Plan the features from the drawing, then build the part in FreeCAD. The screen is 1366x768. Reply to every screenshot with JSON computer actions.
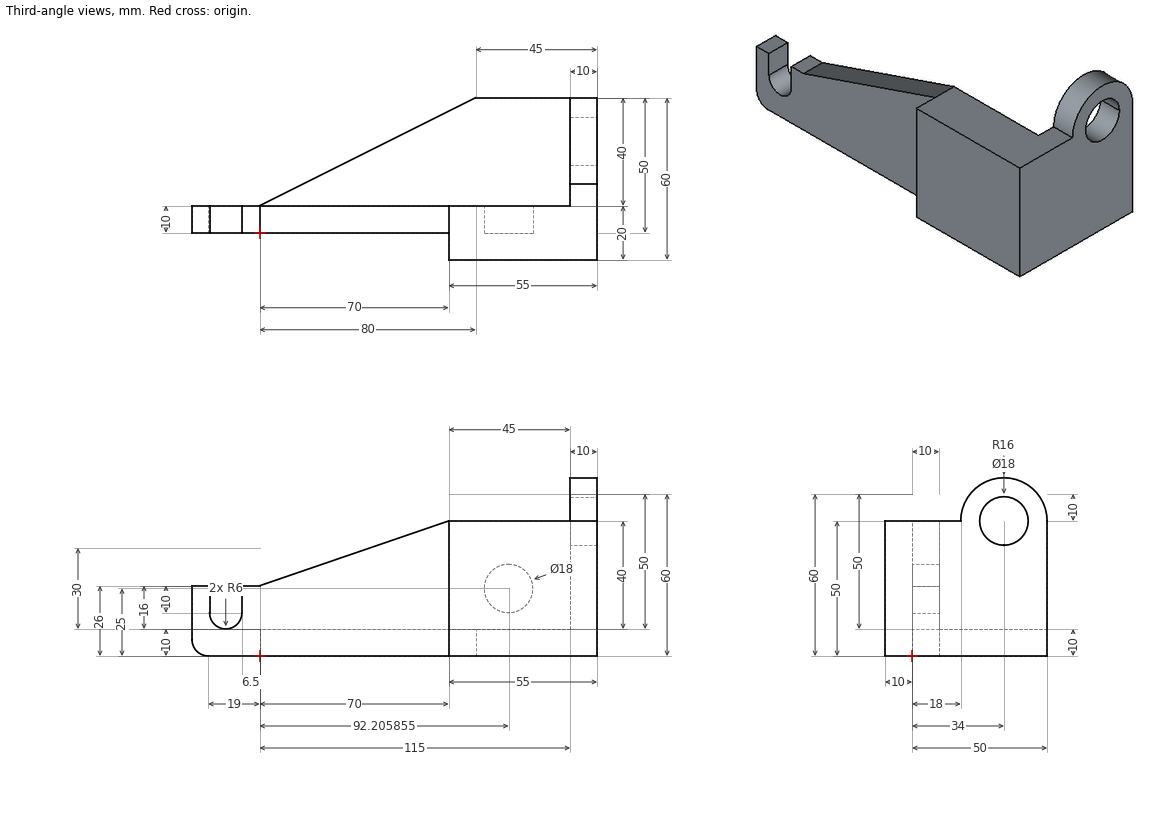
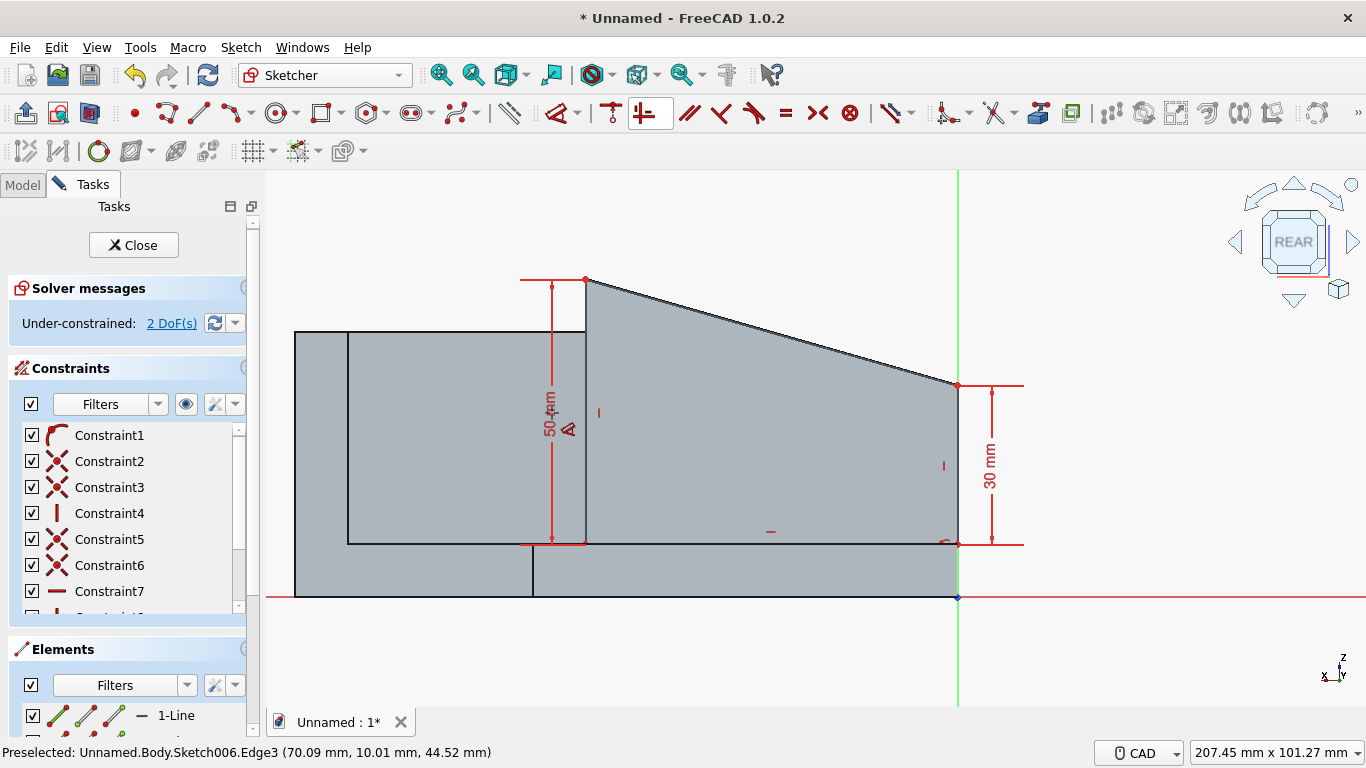
{"action": "left_click", "coordinate": [697, 545]}
{"action": "left_click", "coordinate": [772, 579]}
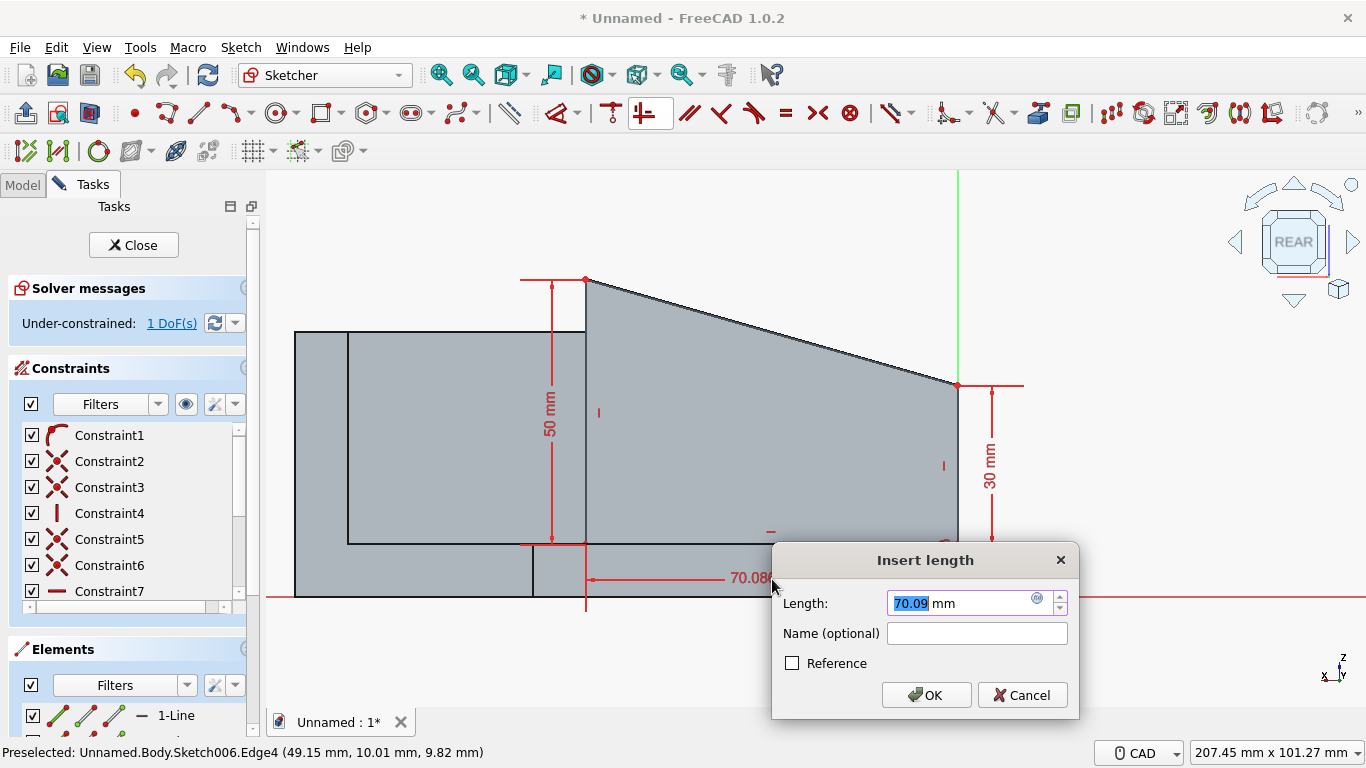
{"action": "type", "text": "70"}
{"action": "key", "text": "Return"}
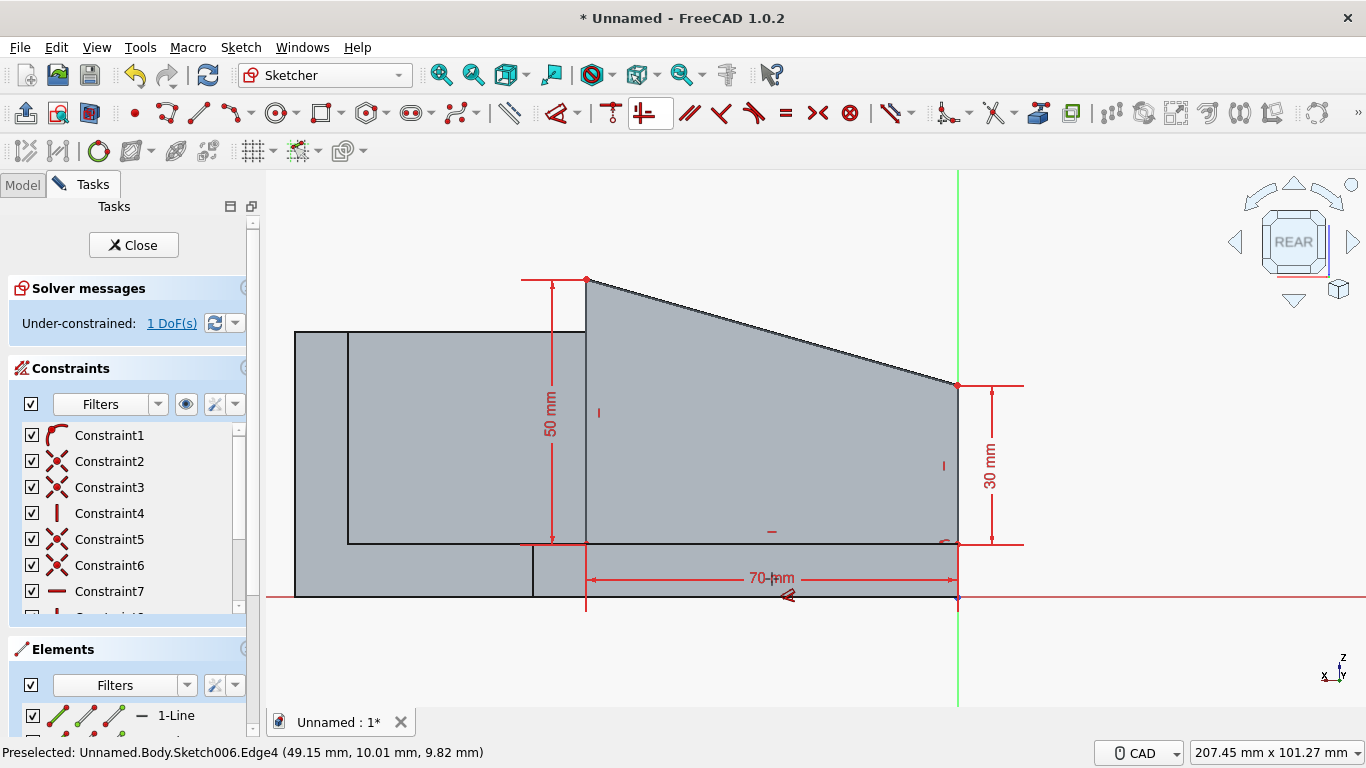
{"action": "left_click", "coordinate": [958, 545]}
{"action": "left_click", "coordinate": [992, 571]}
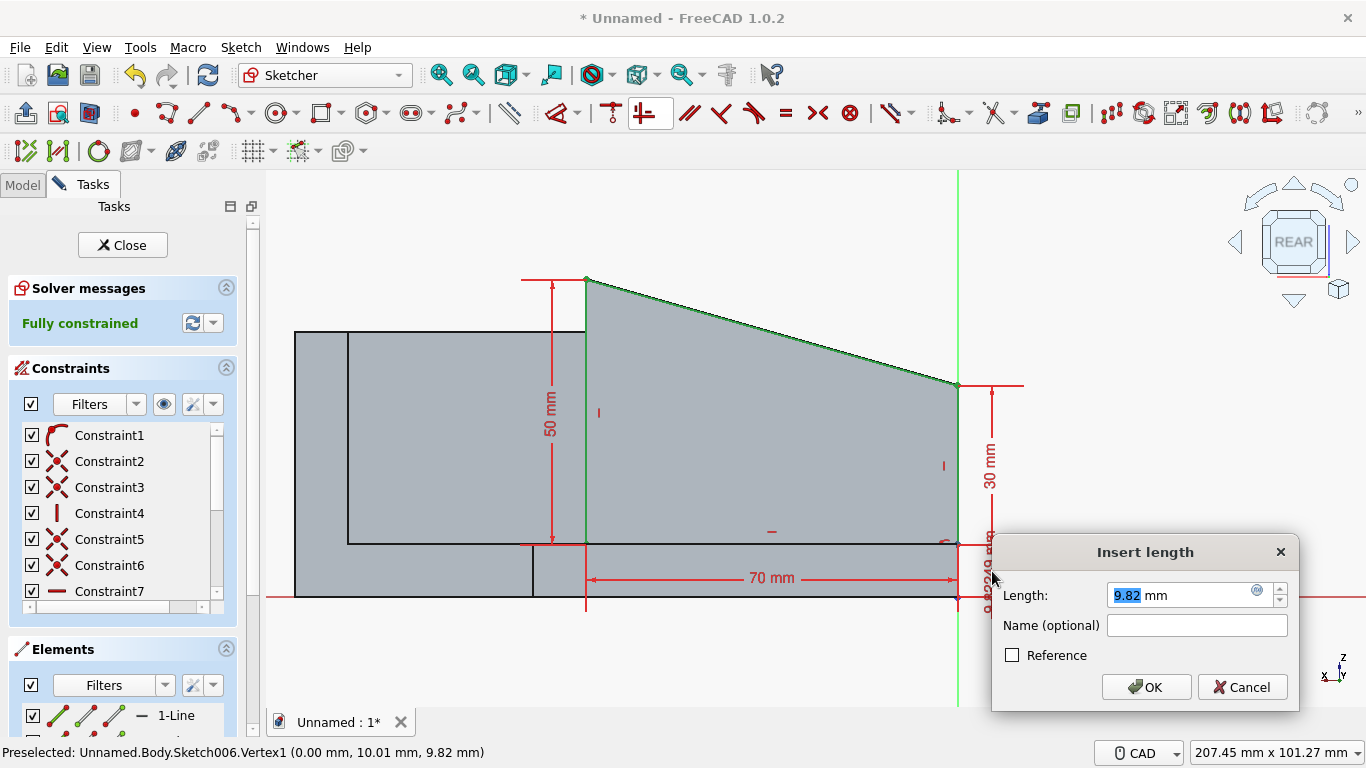
{"action": "type", "text": "10"}
{"action": "key", "text": "Return"}
{"action": "key", "text": "Escape"}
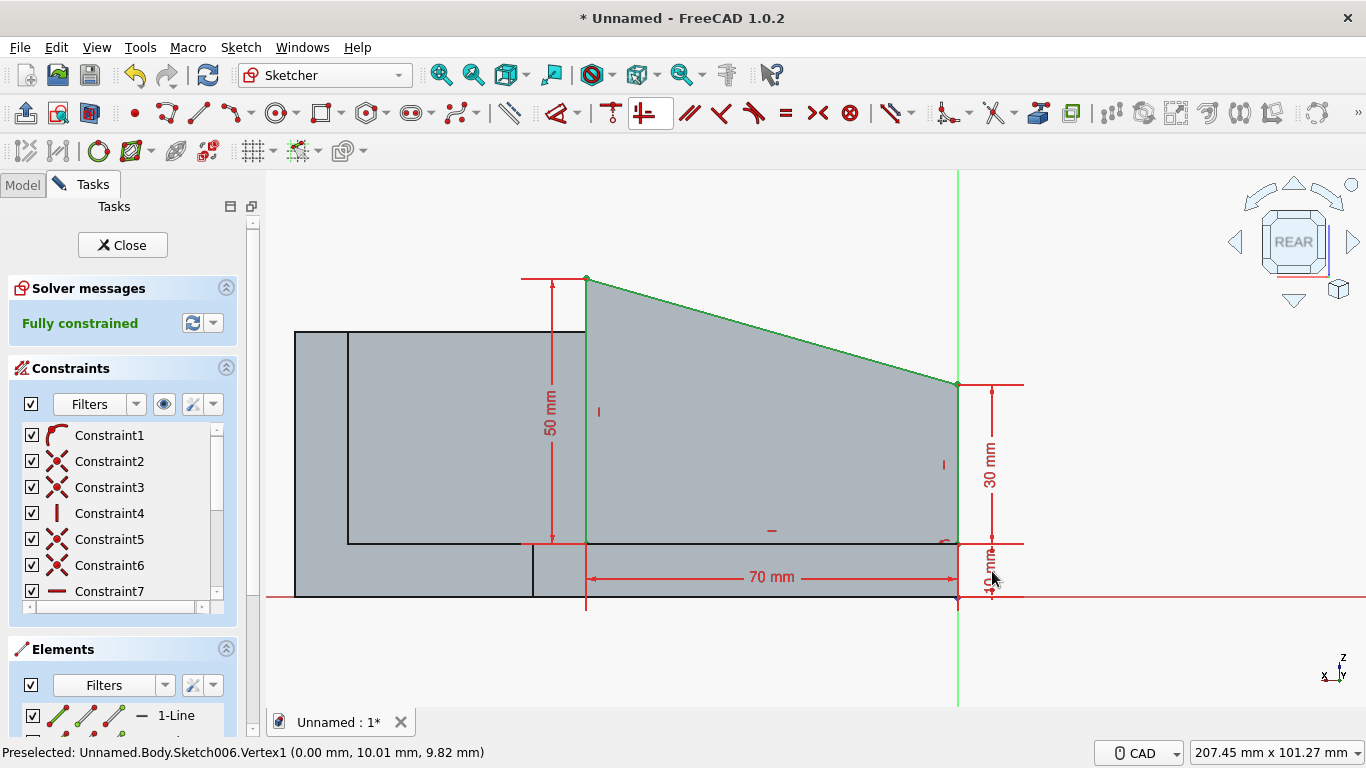
{"action": "left_click", "coordinate": [123, 245]}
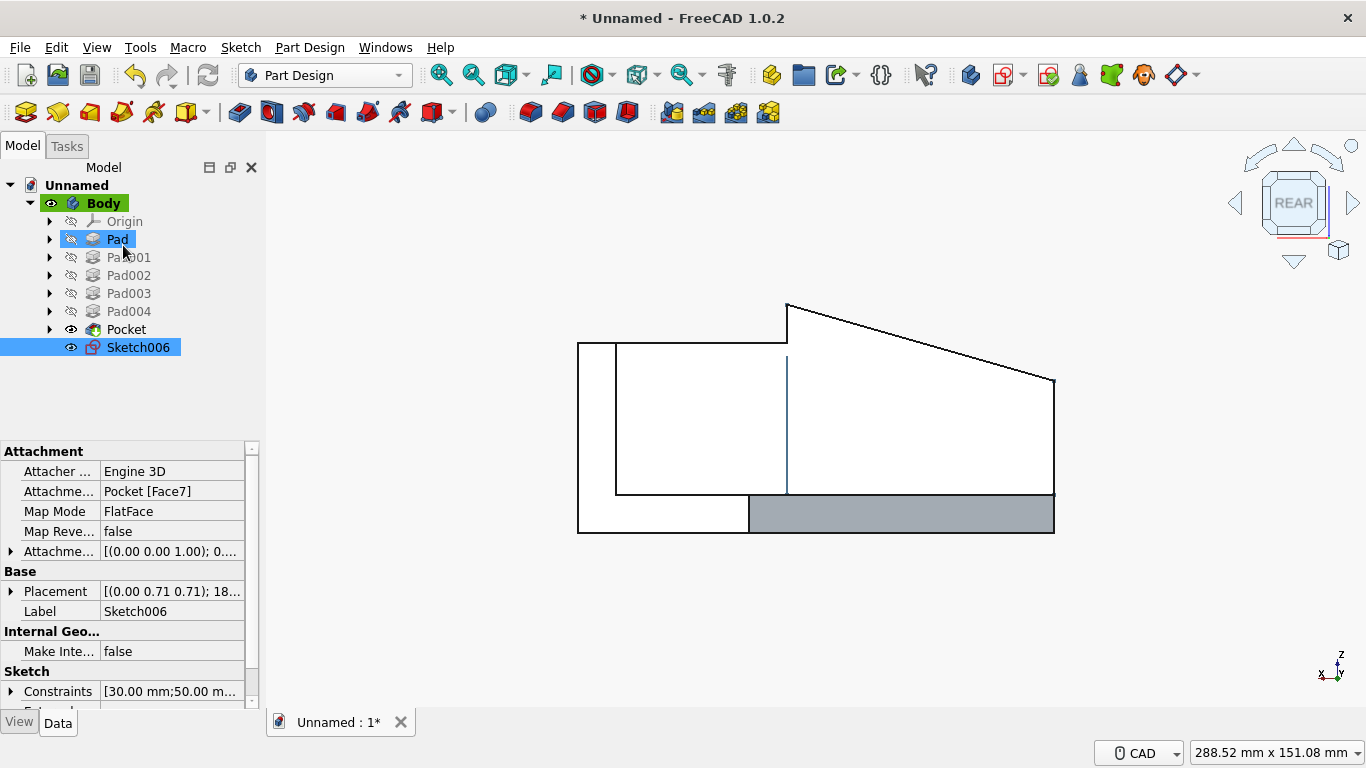
{"action": "left_click", "coordinate": [240, 112]}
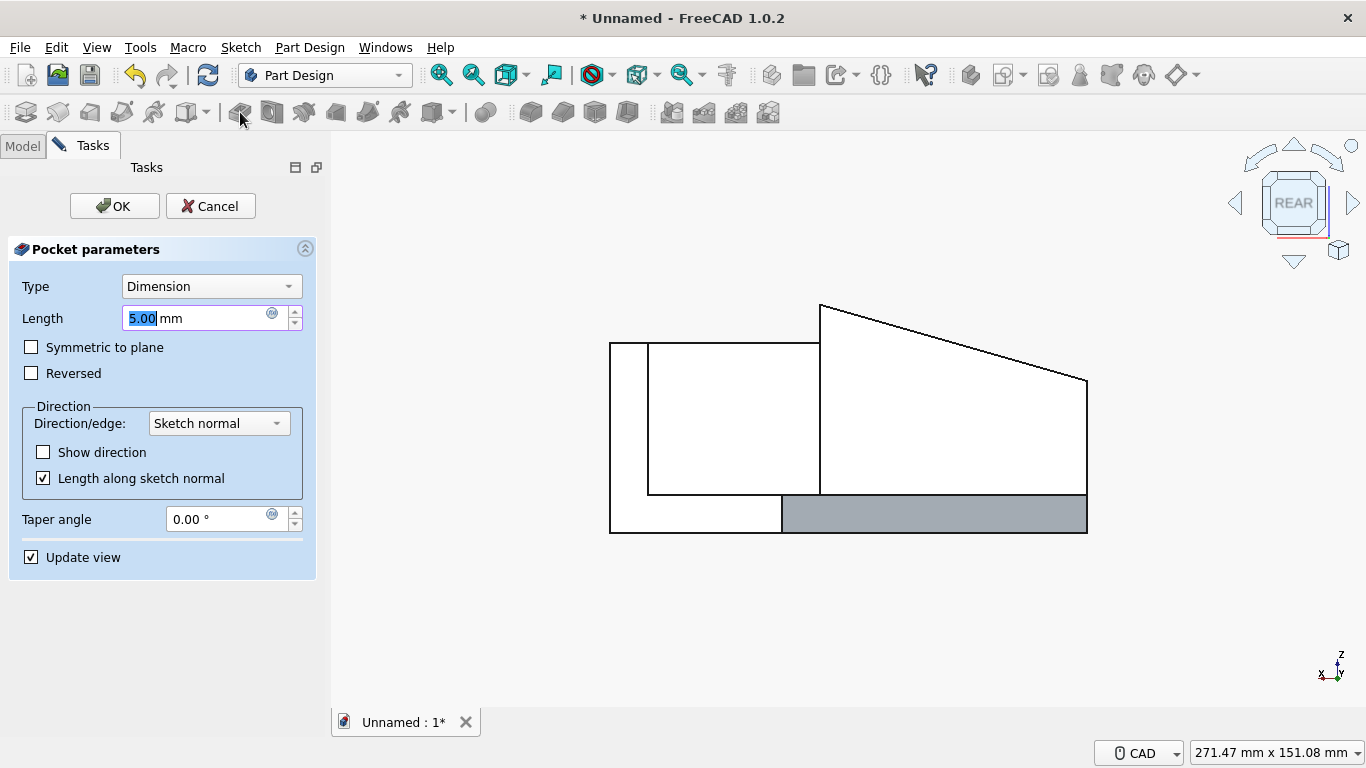
{"action": "type", "text": "10"}
{"action": "key", "text": "Tab"}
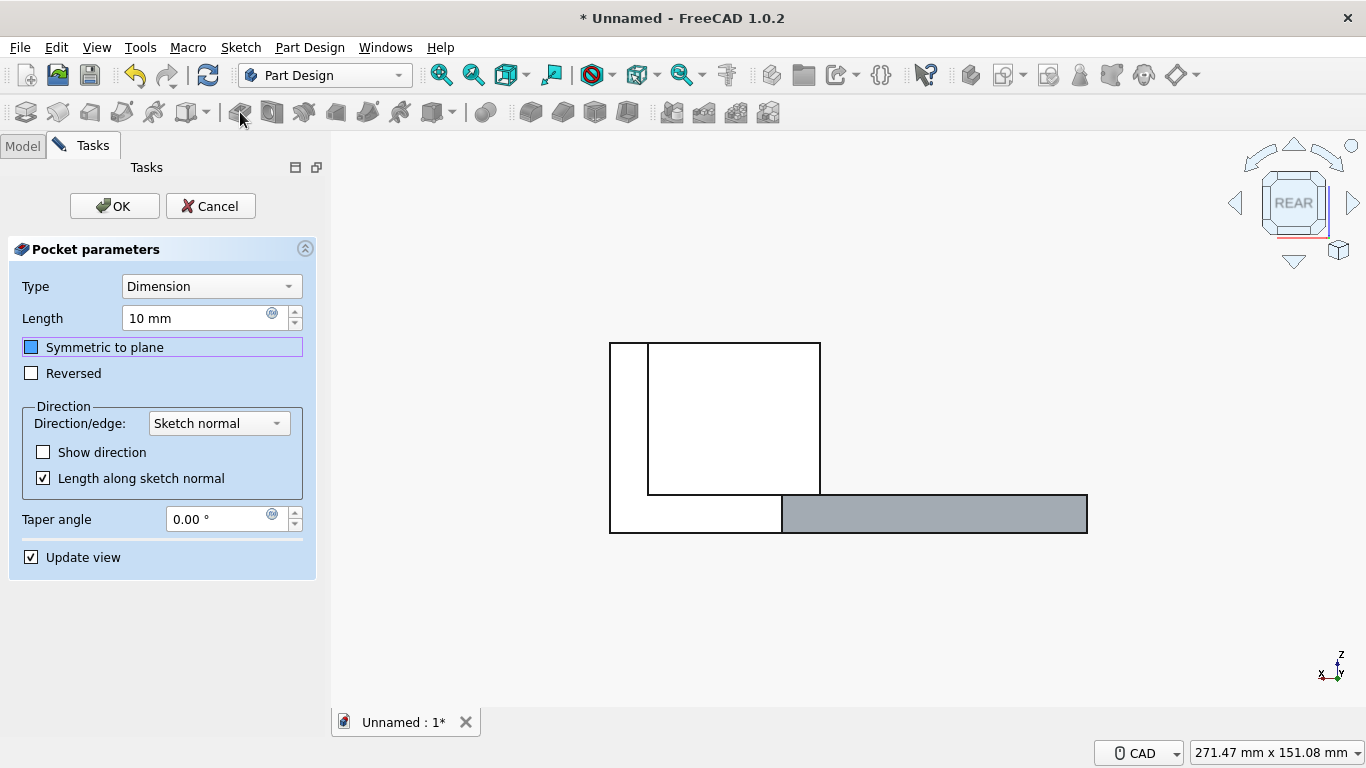
{"action": "left_click", "coordinate": [115, 206]}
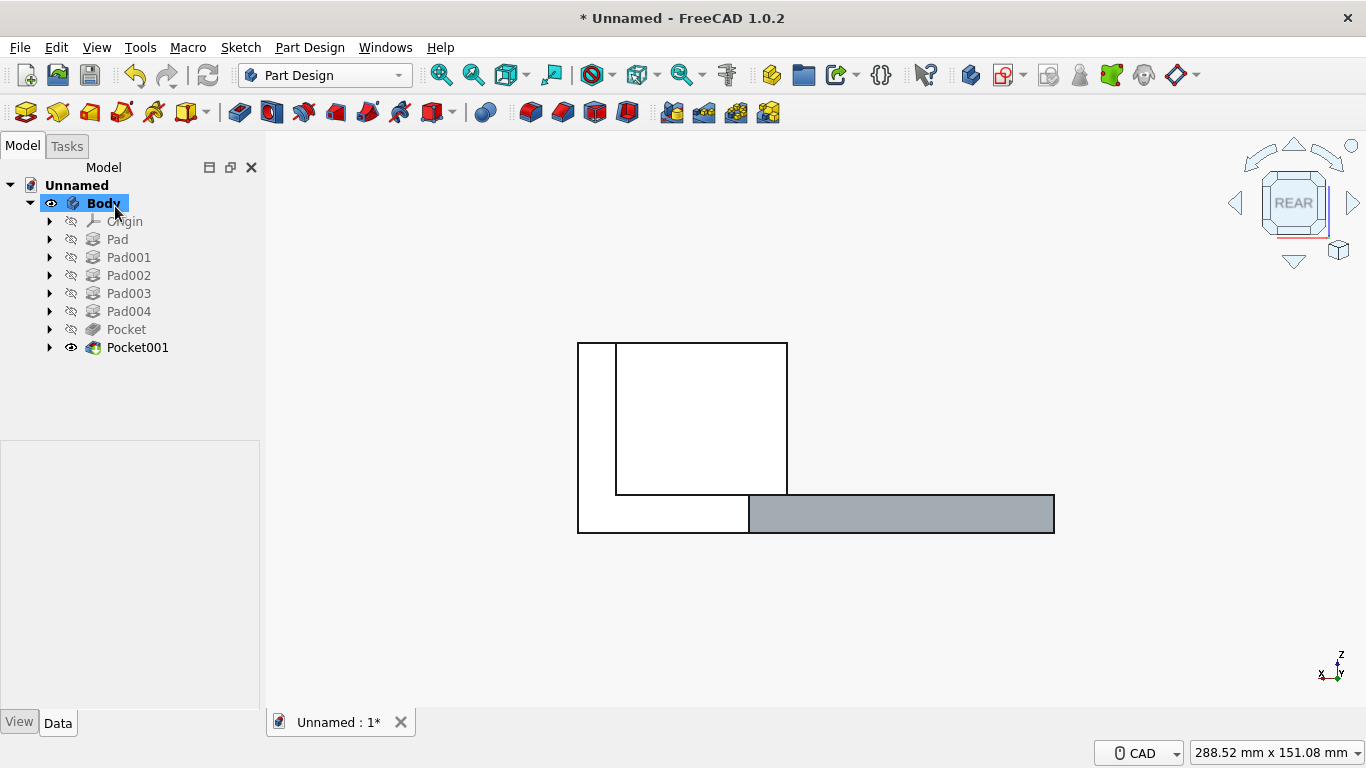
{"action": "left_click", "coordinate": [442, 76]}